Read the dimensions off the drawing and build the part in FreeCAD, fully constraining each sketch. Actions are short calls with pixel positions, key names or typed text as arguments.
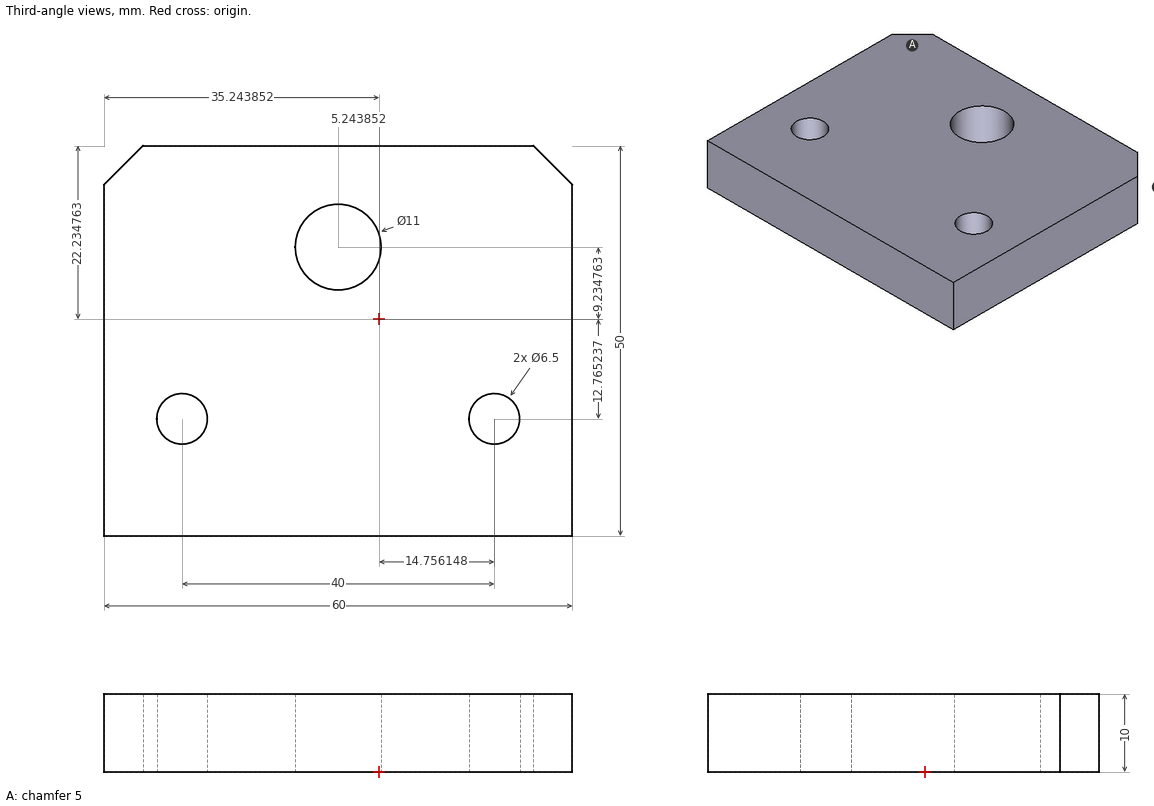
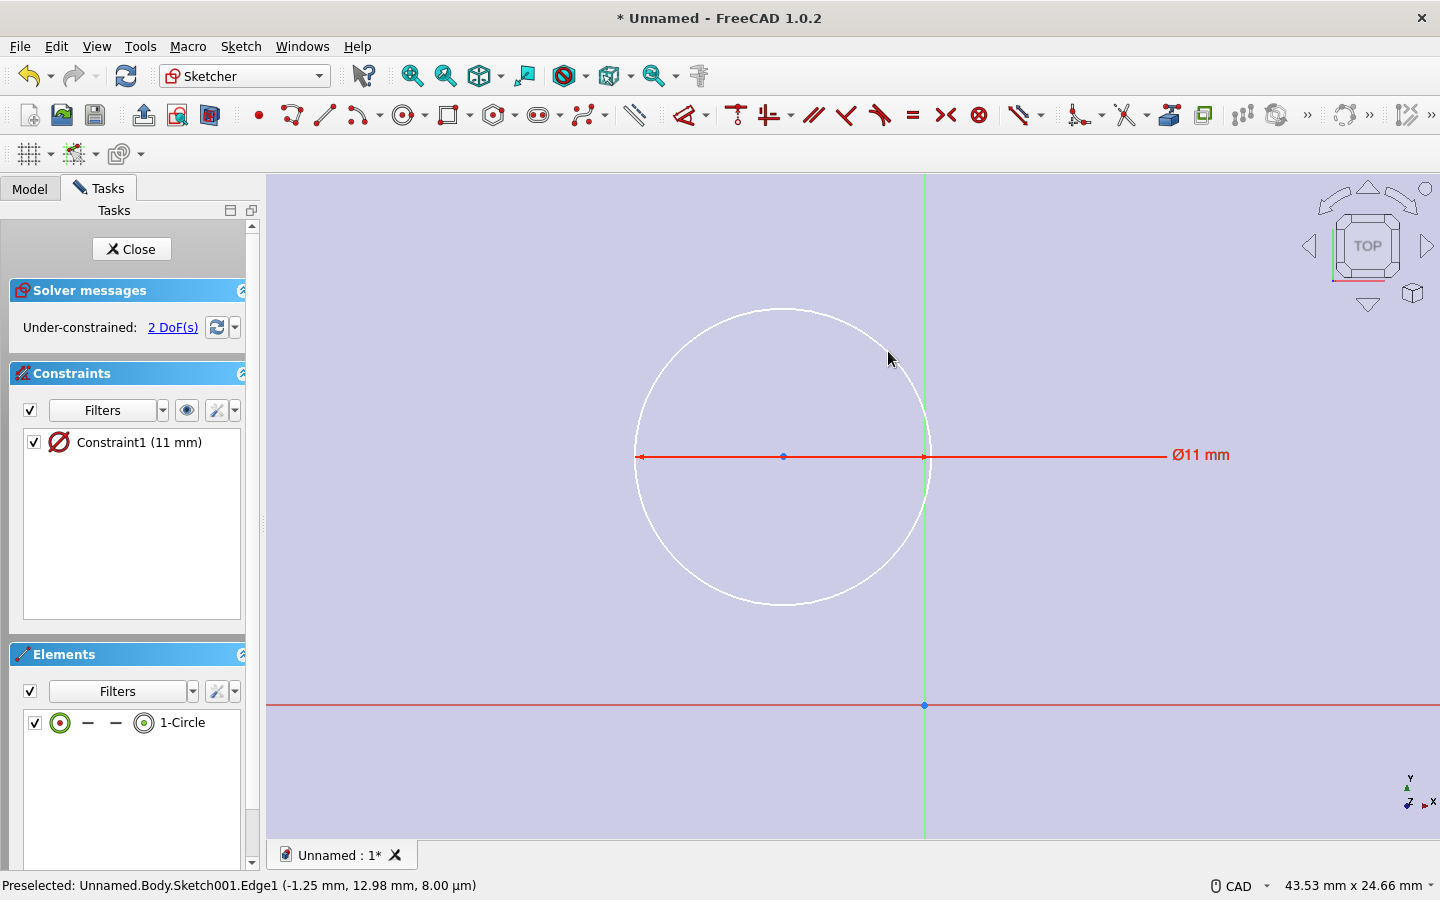
key(d)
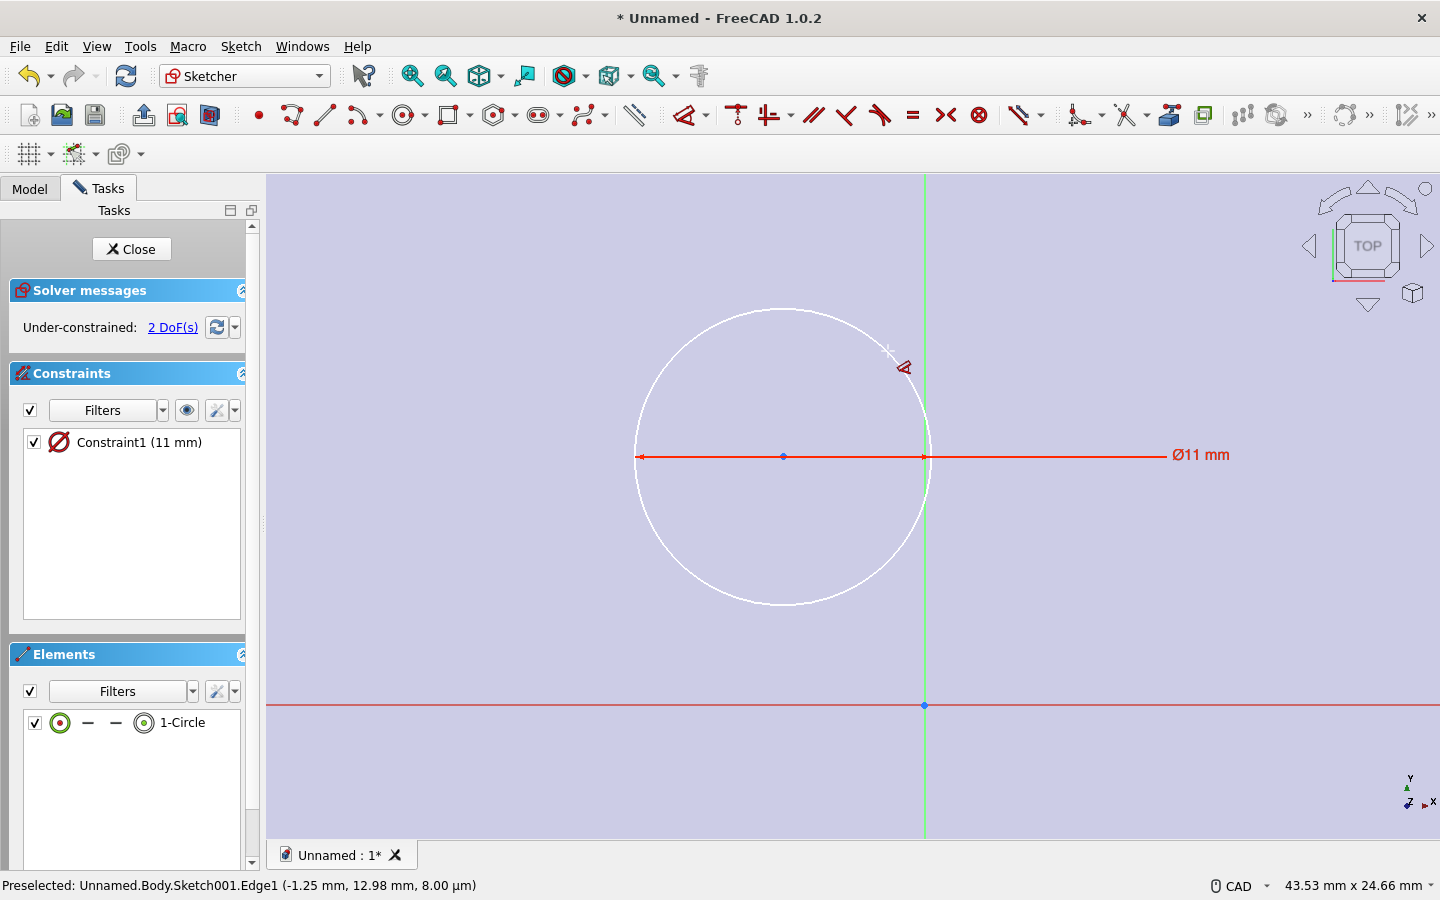
click(783, 457)
click(854, 739)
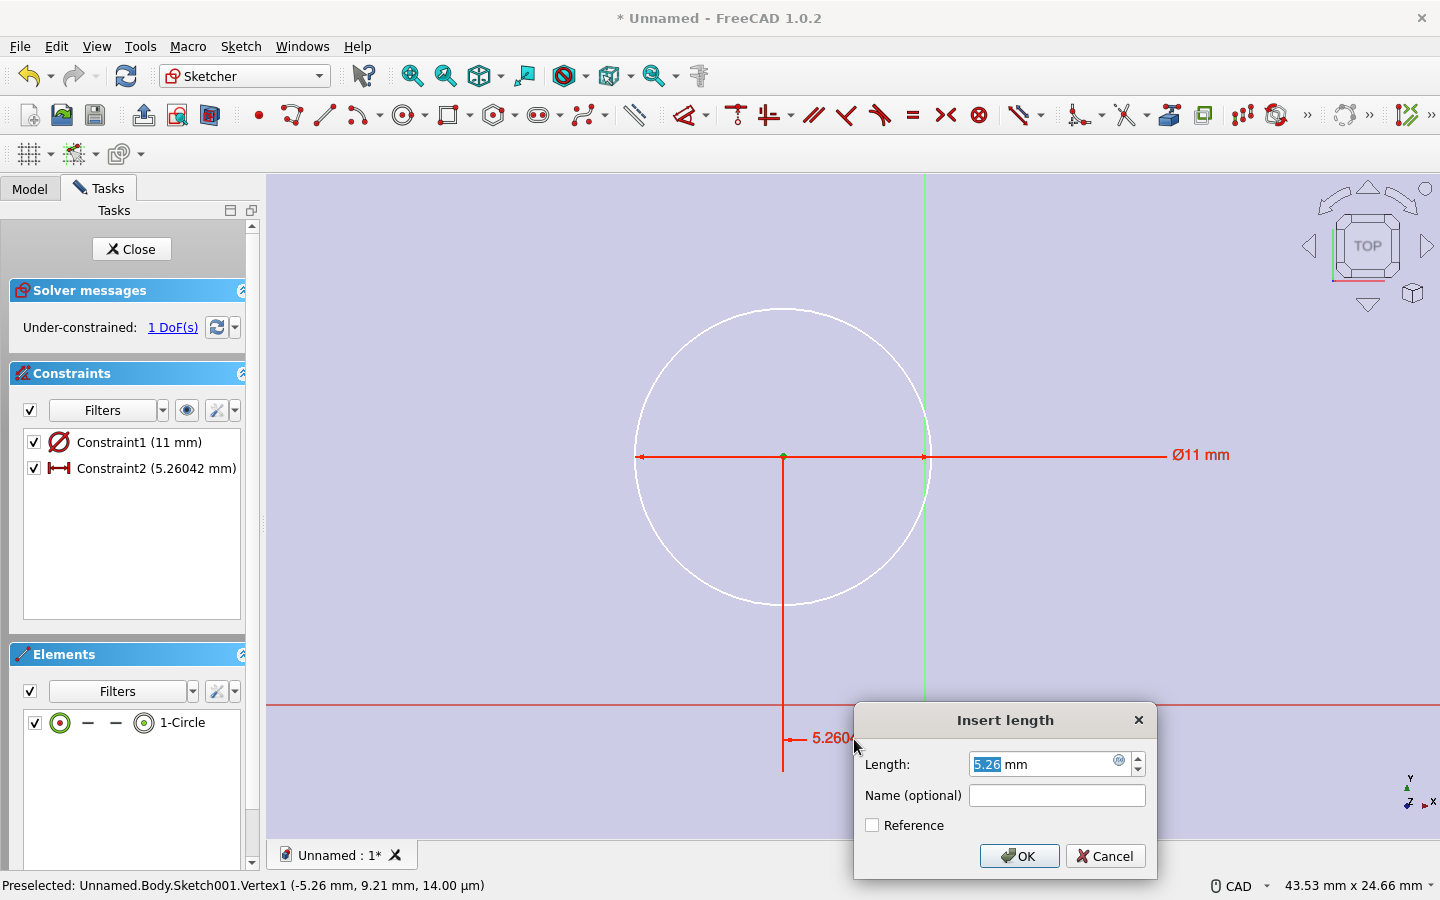
text(5.243852)
key(Return)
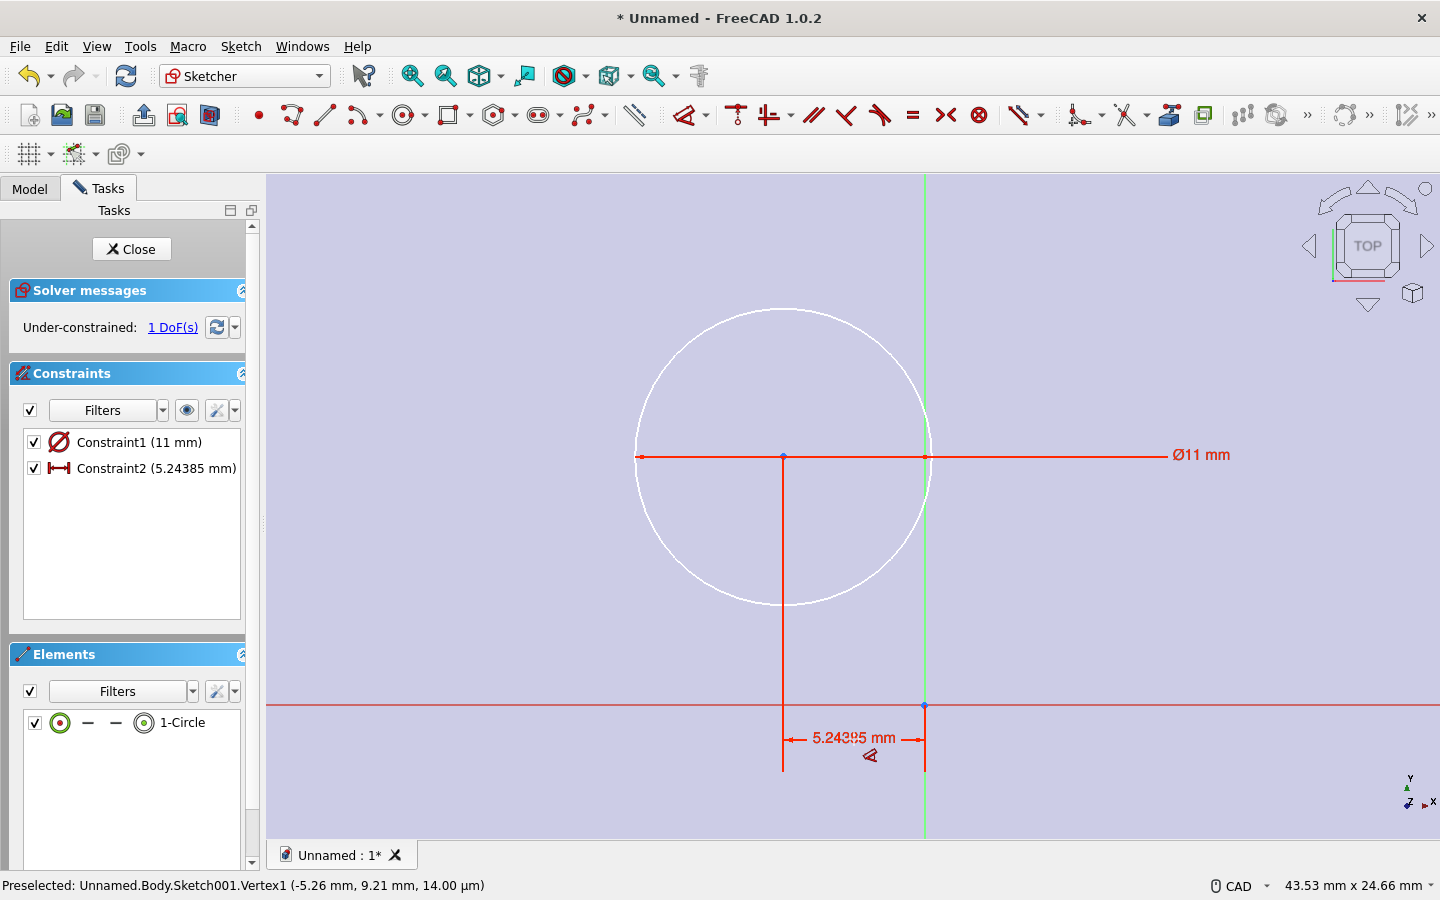
click(783, 457)
click(959, 581)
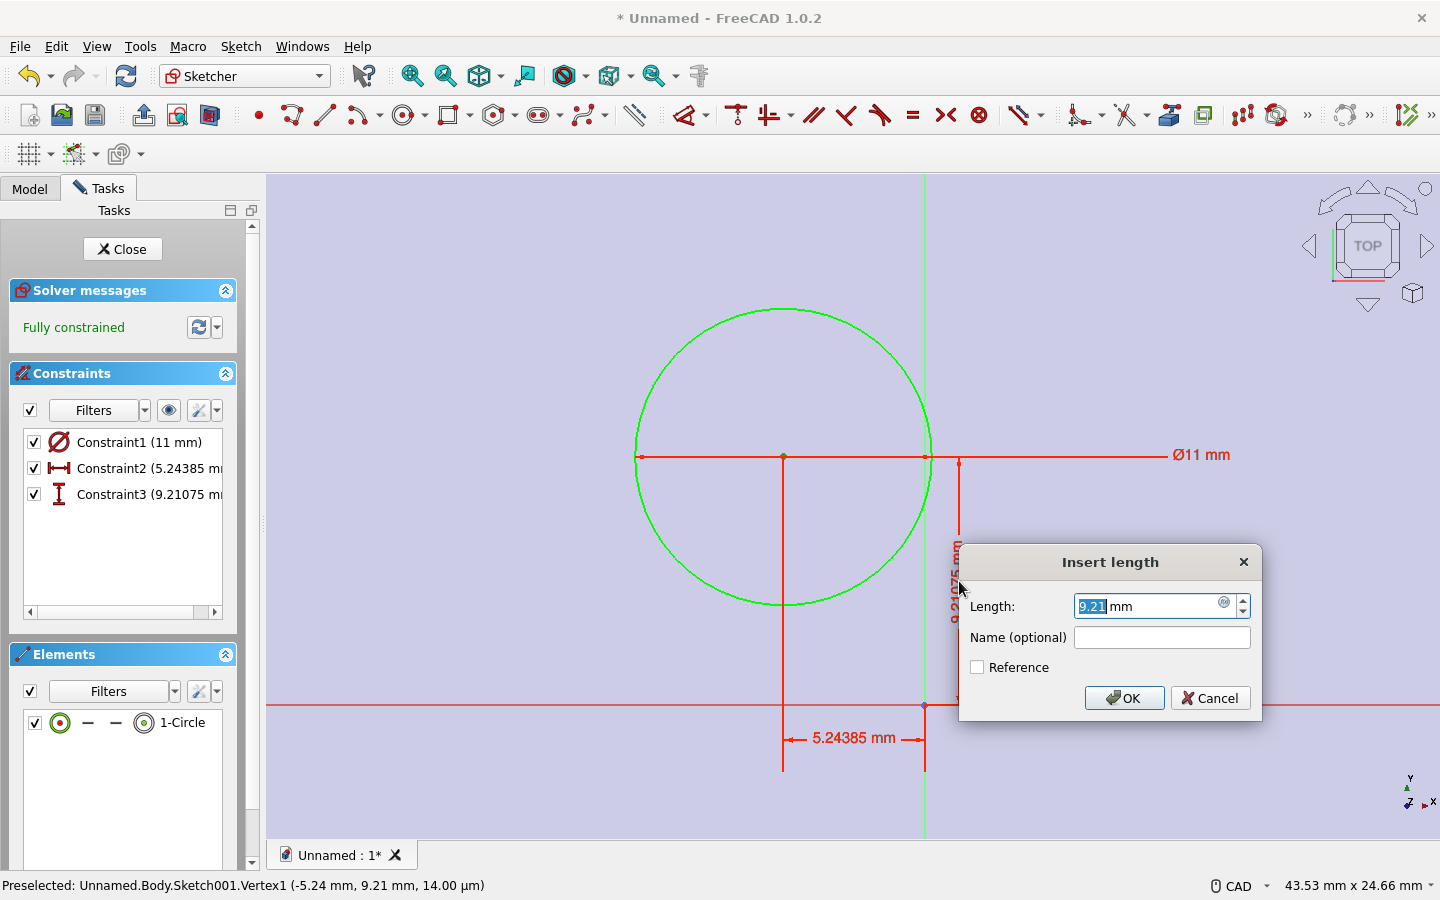
text(9.234763)
key(Return)
key(Escape)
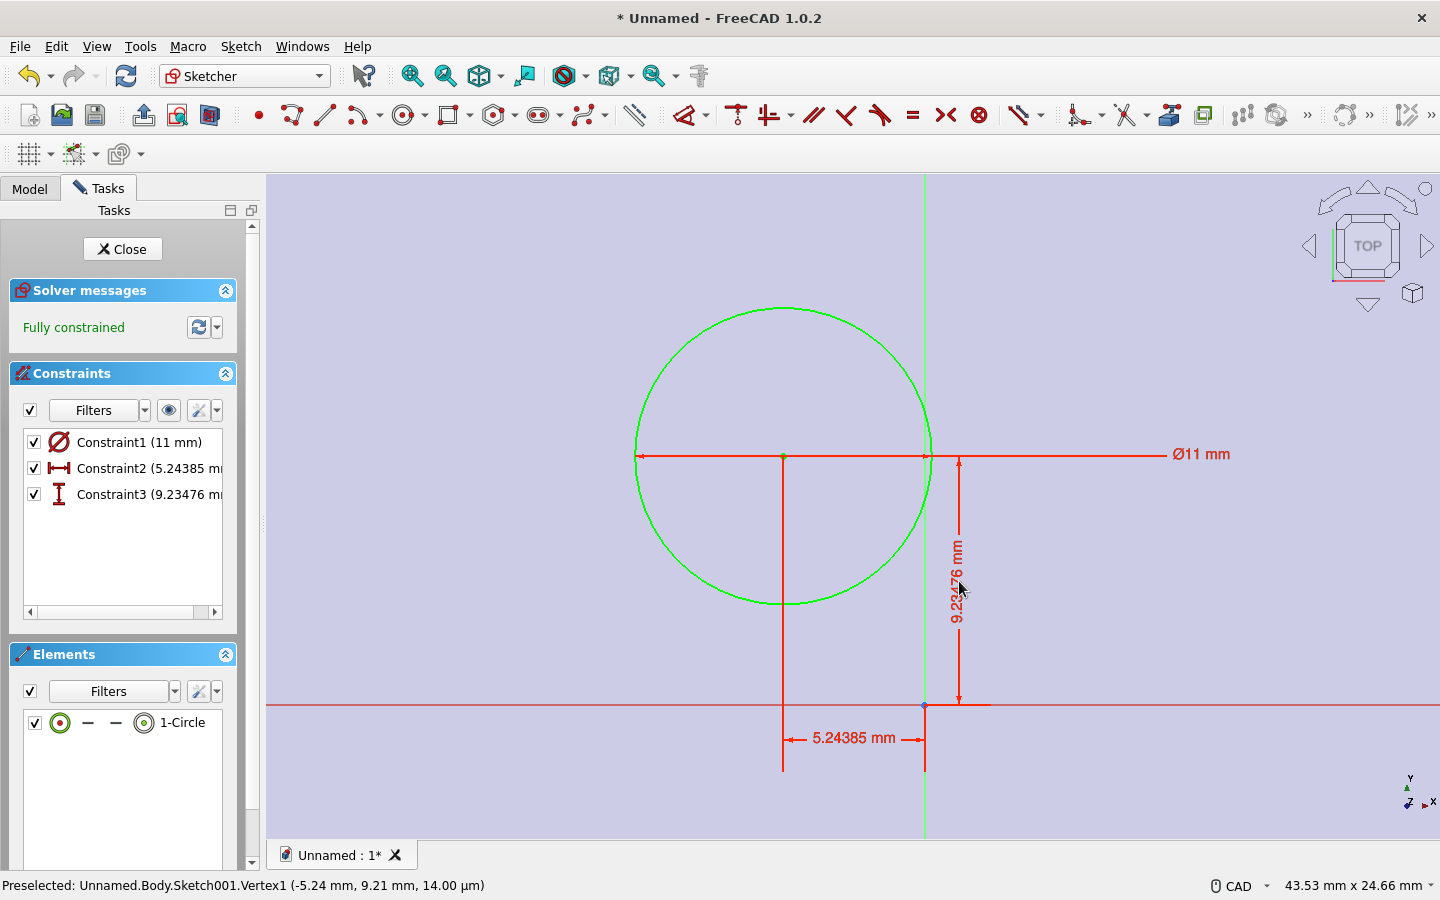
click(123, 249)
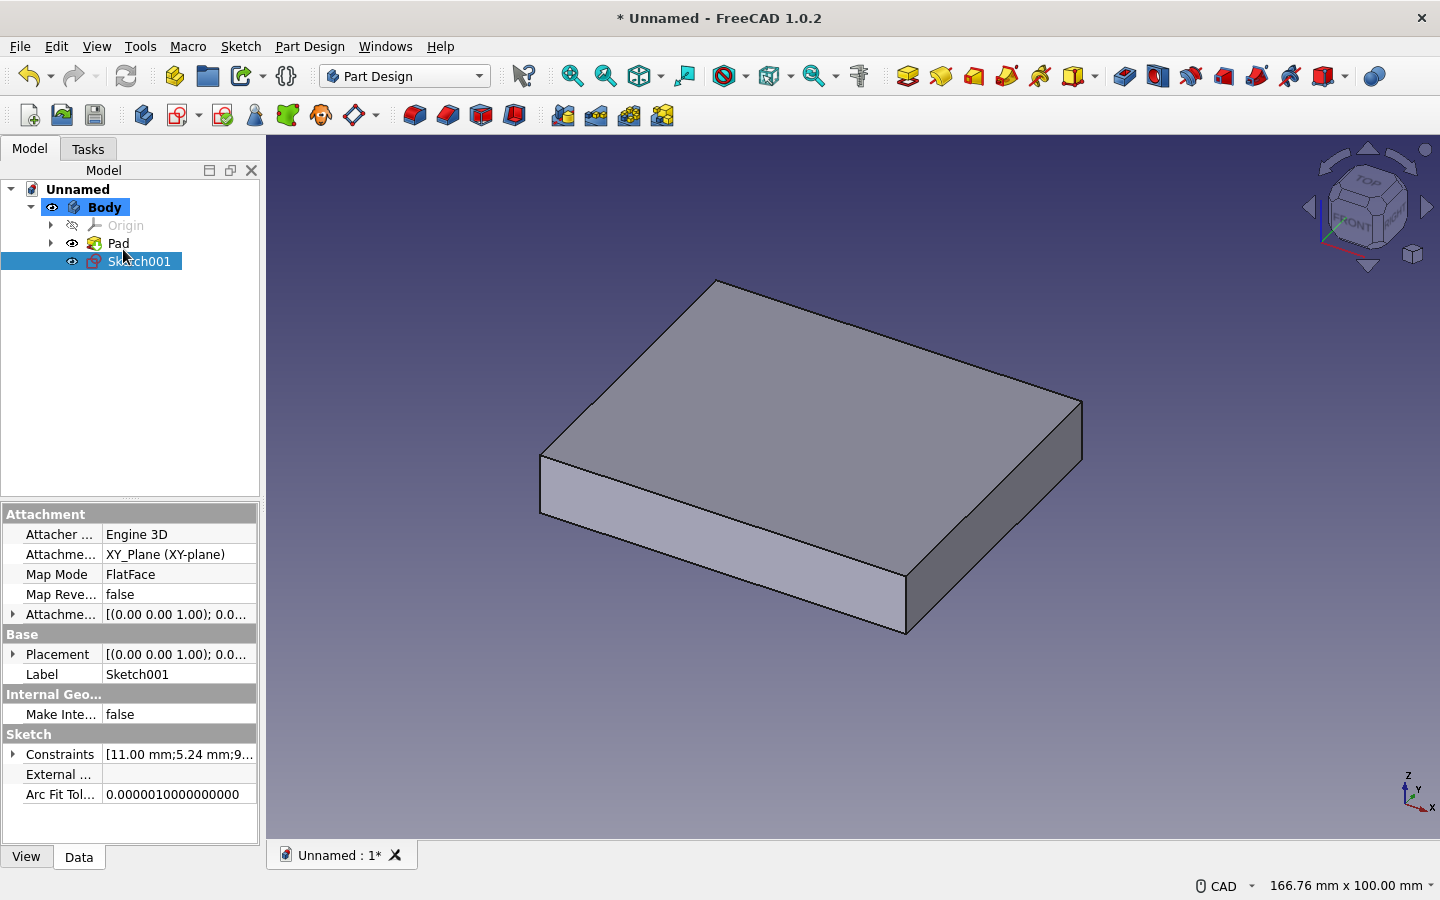
click(1125, 76)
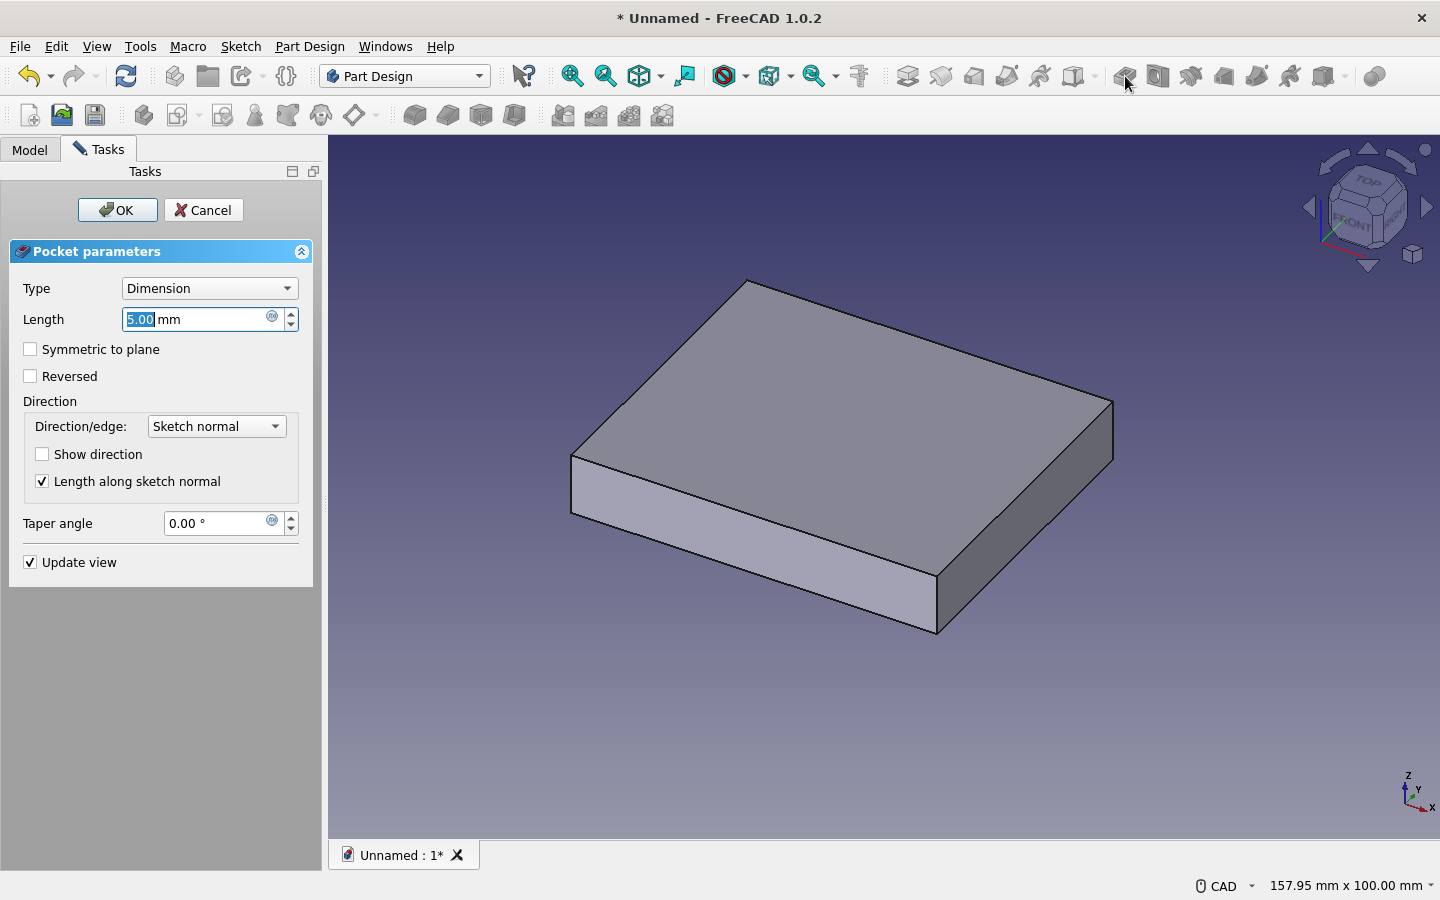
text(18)
key(Tab)